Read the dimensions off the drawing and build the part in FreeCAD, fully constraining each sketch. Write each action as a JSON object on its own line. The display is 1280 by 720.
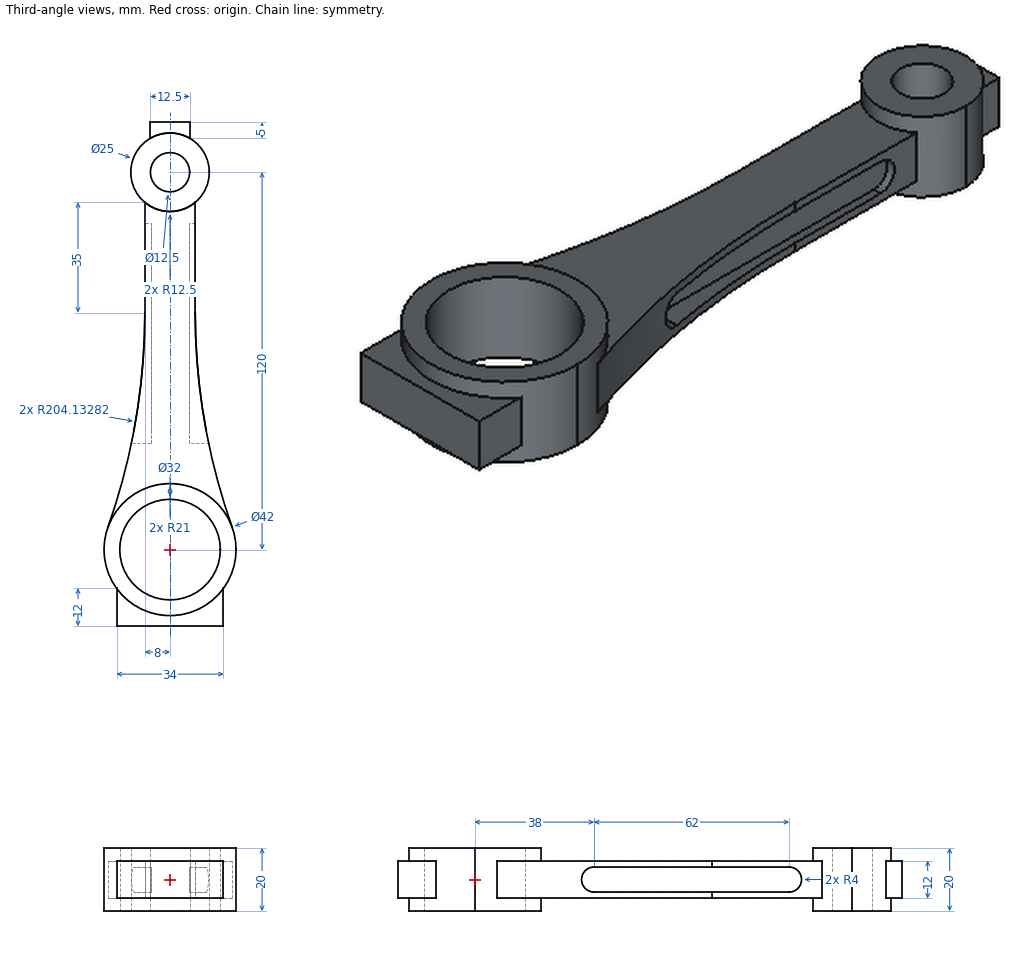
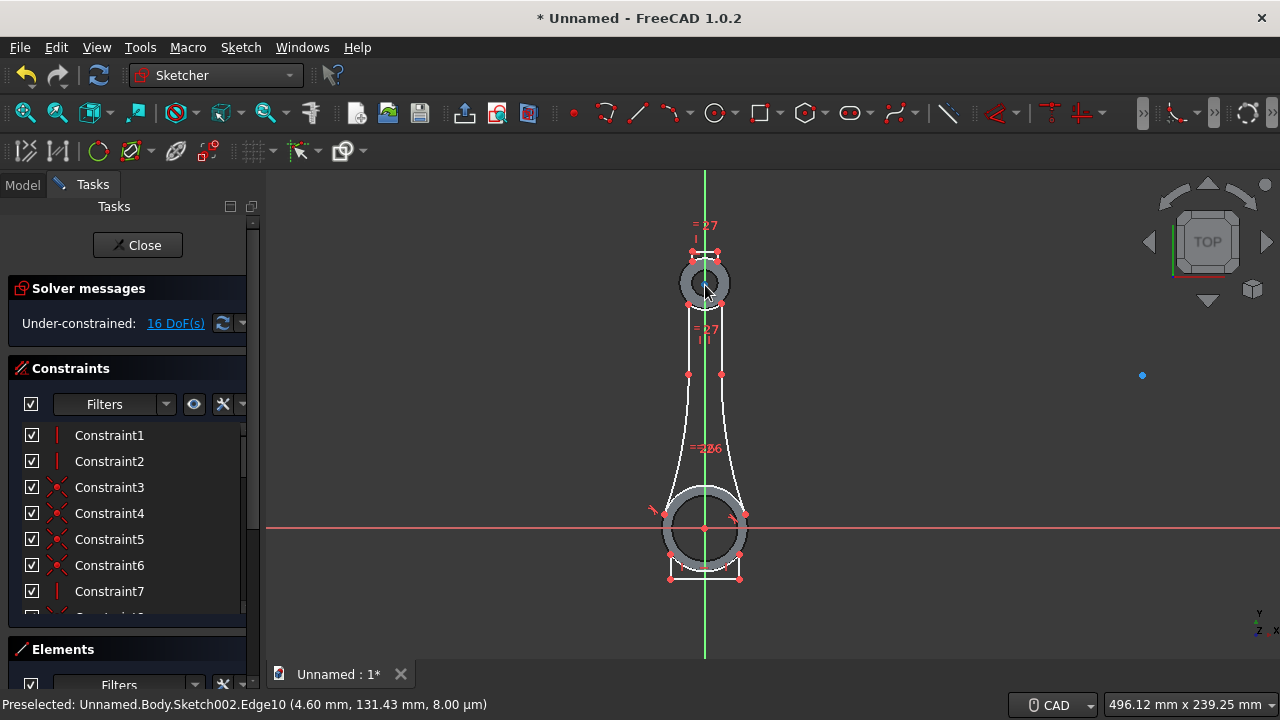
{"action": "left_click", "coordinate": [725, 491]}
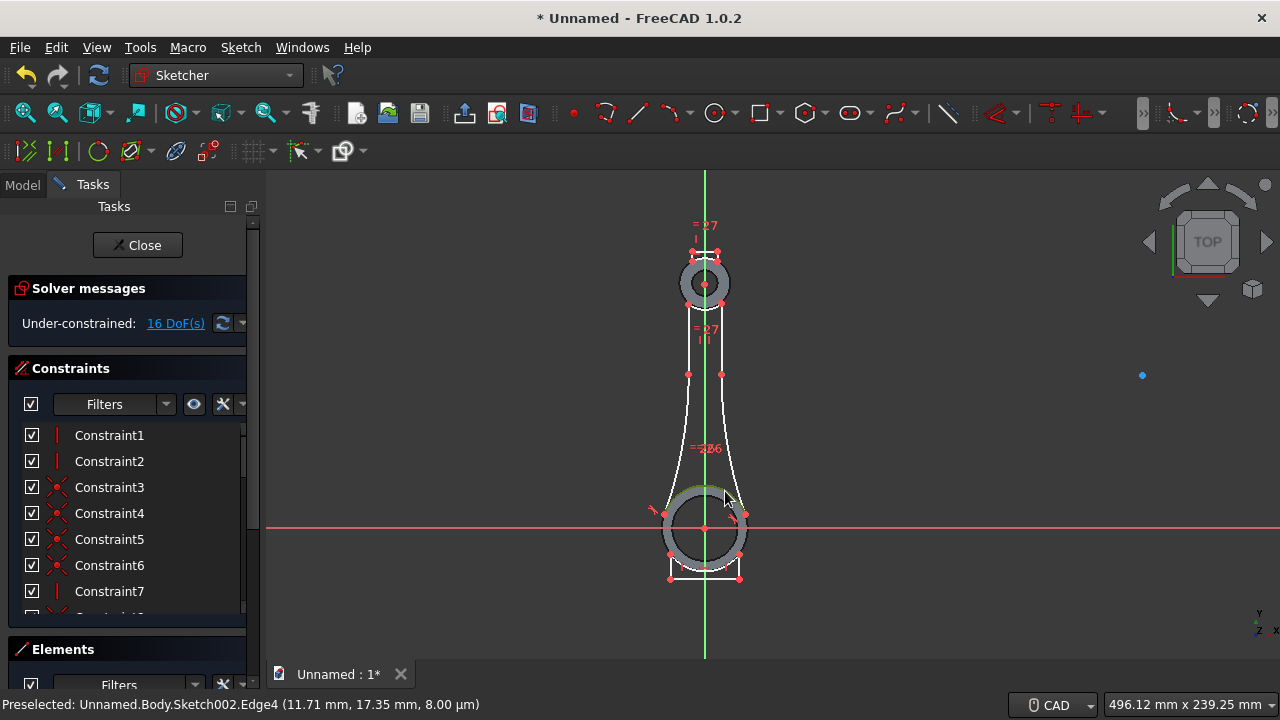
{"action": "scroll", "coordinate": [689, 569], "scroll_direction": "up", "scroll_amount": 2}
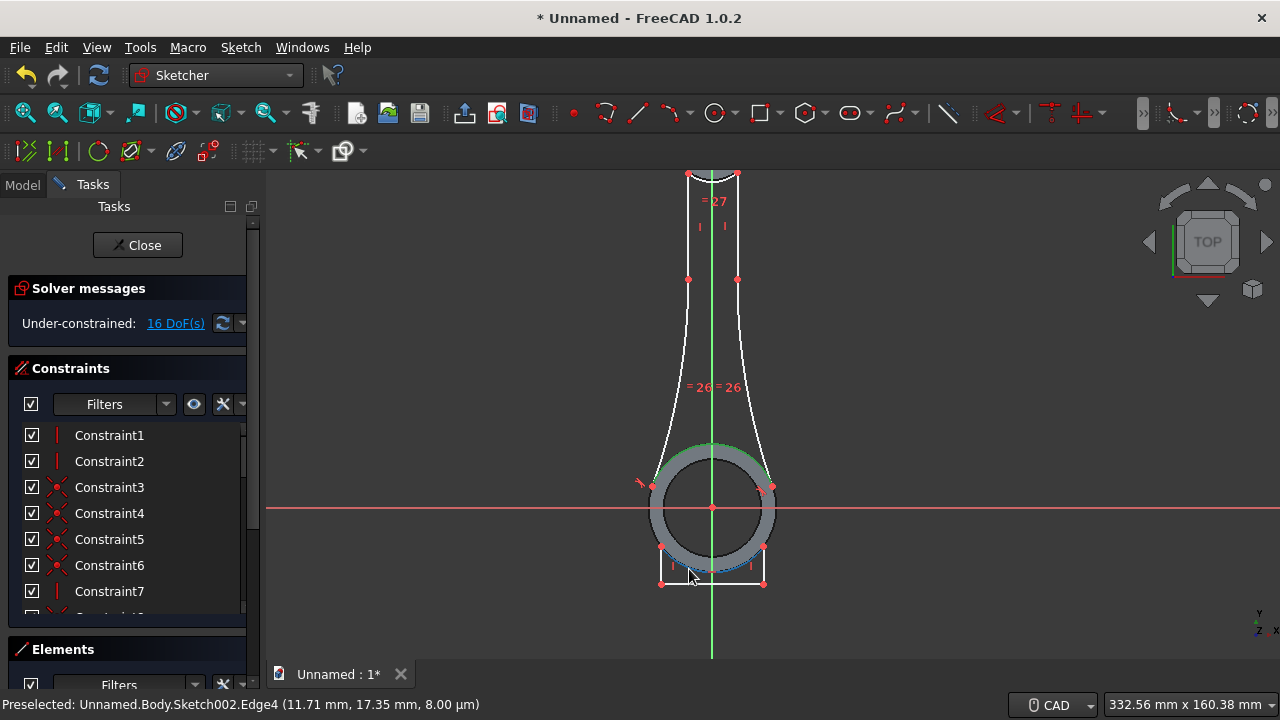
{"action": "left_click", "coordinate": [689, 568]}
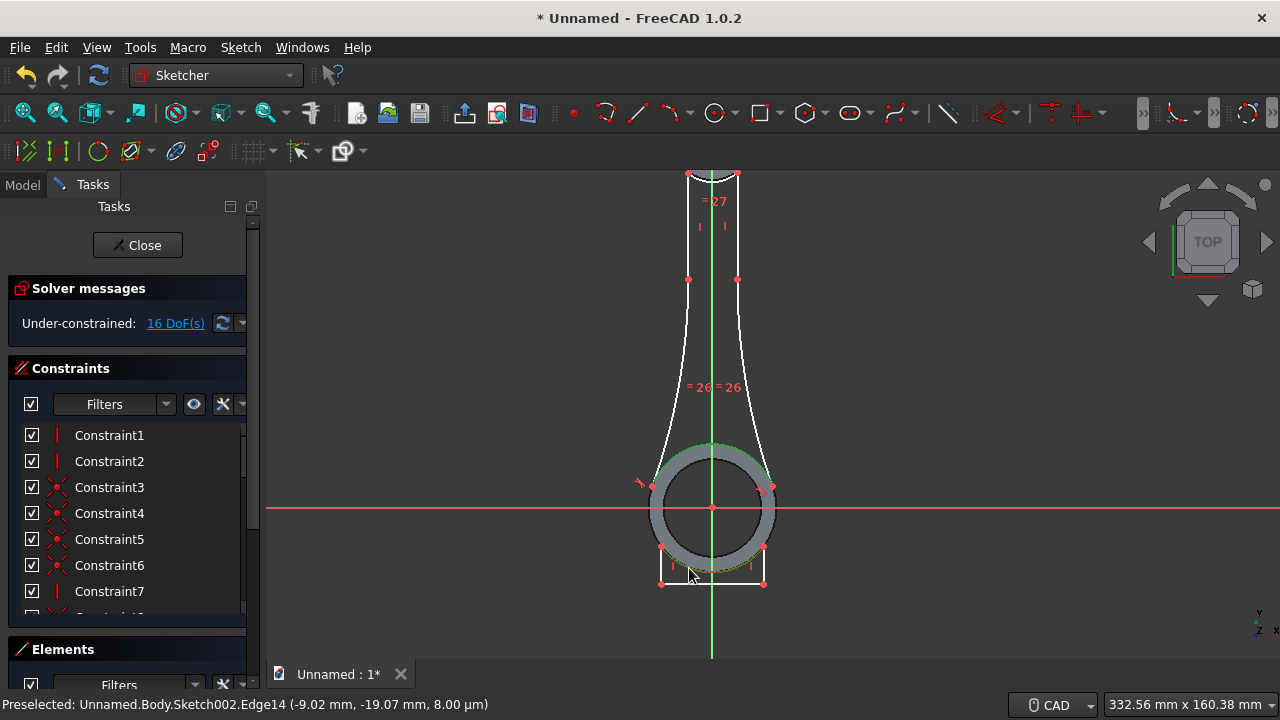
{"action": "key", "text": "e"}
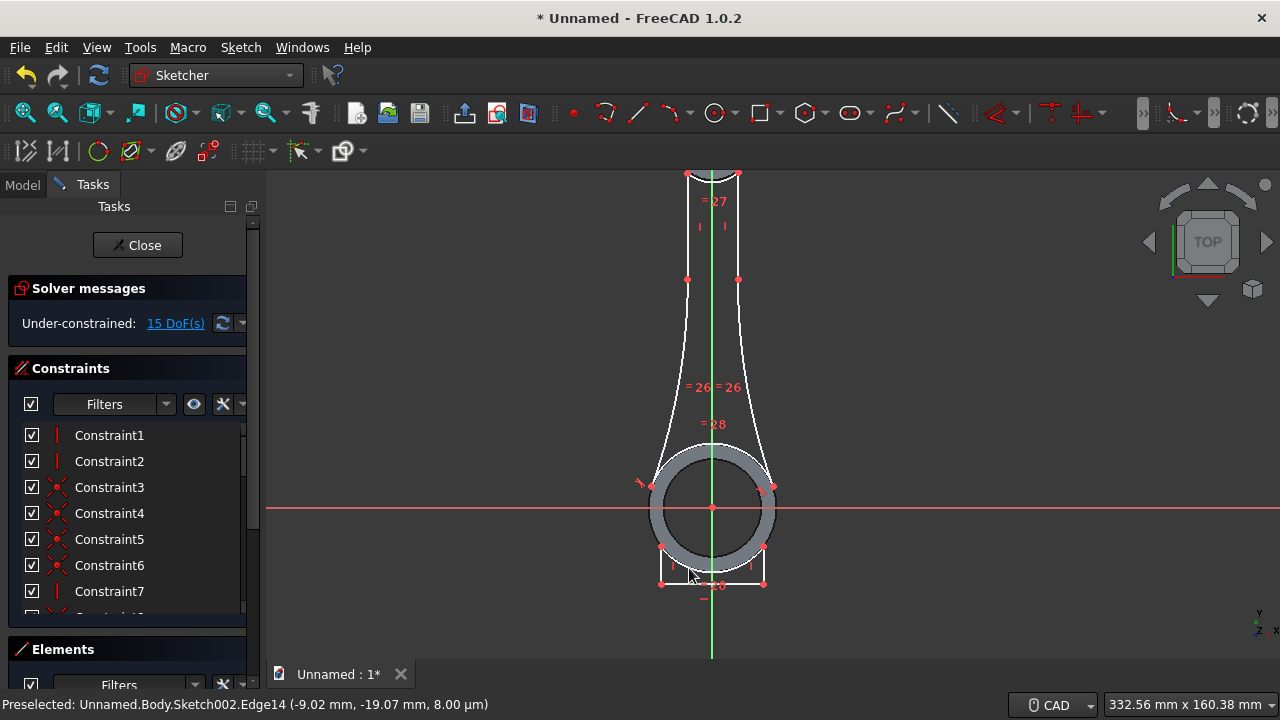
{"action": "scroll", "coordinate": [688, 570], "scroll_direction": "down", "scroll_amount": 2}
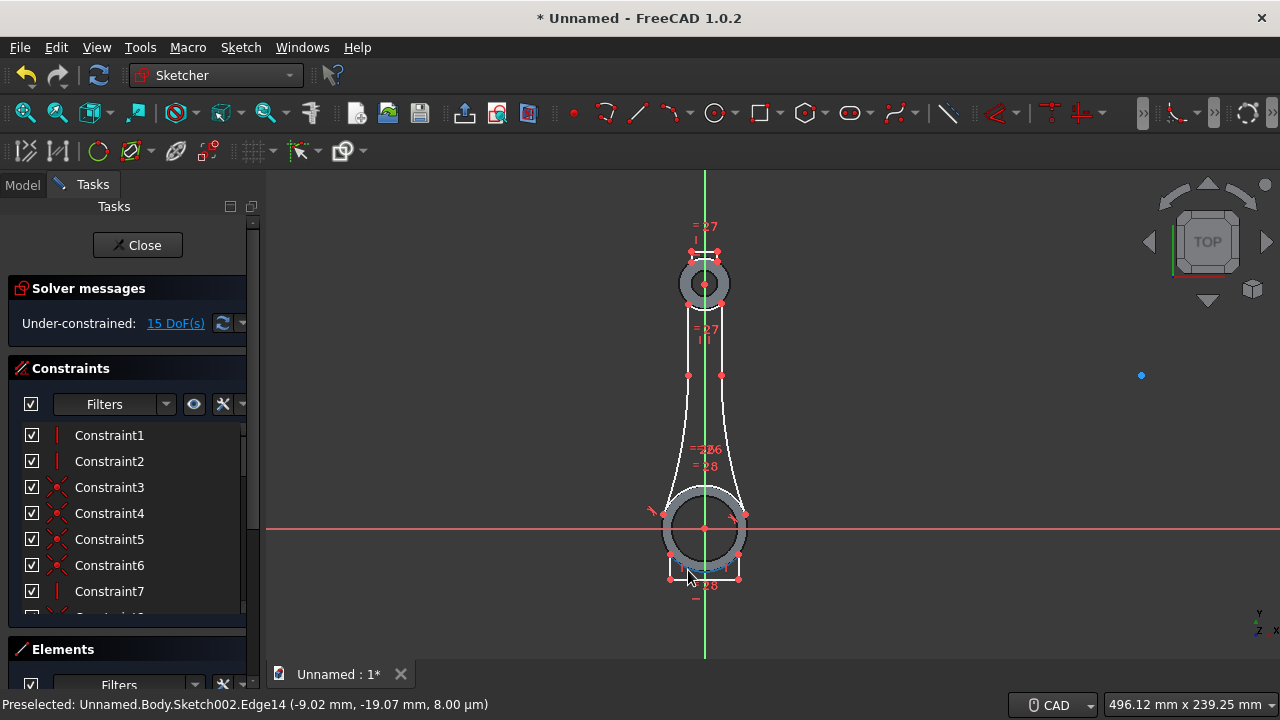
{"action": "left_click", "coordinate": [705, 285]}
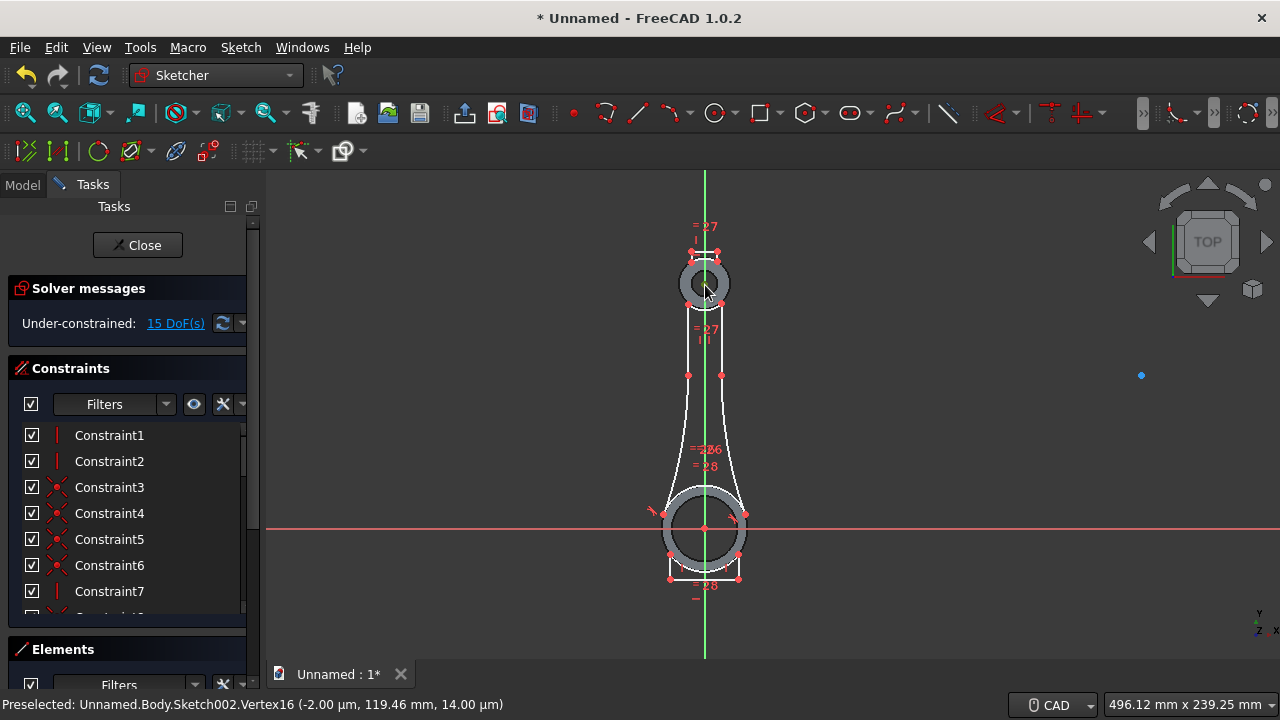
{"action": "left_click", "coordinate": [705, 507]}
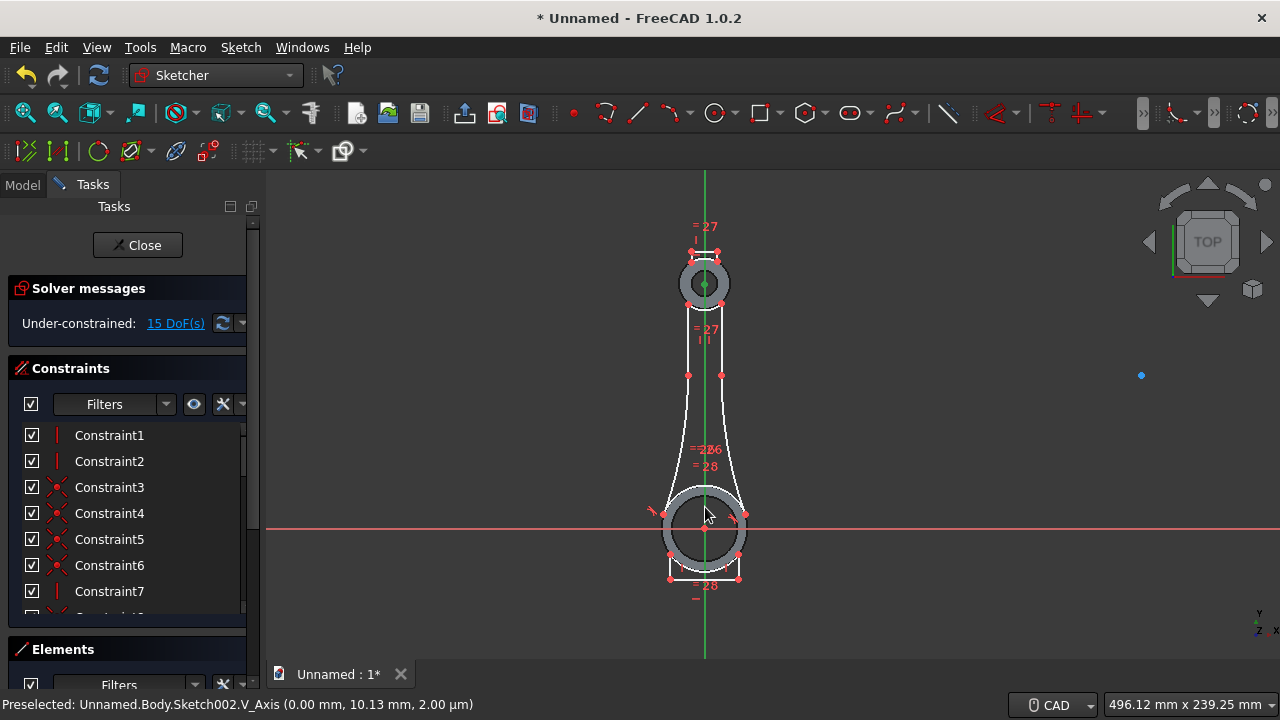
{"action": "key", "text": "c"}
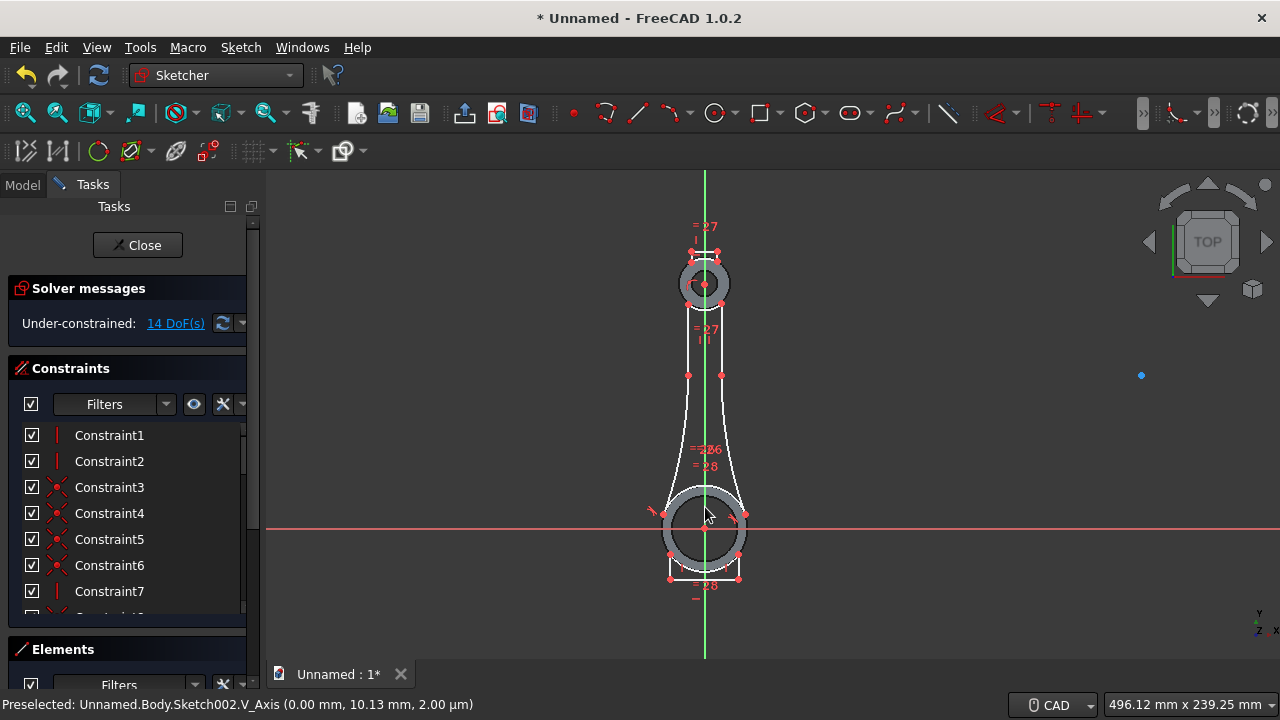
{"action": "left_click", "coordinate": [688, 375]}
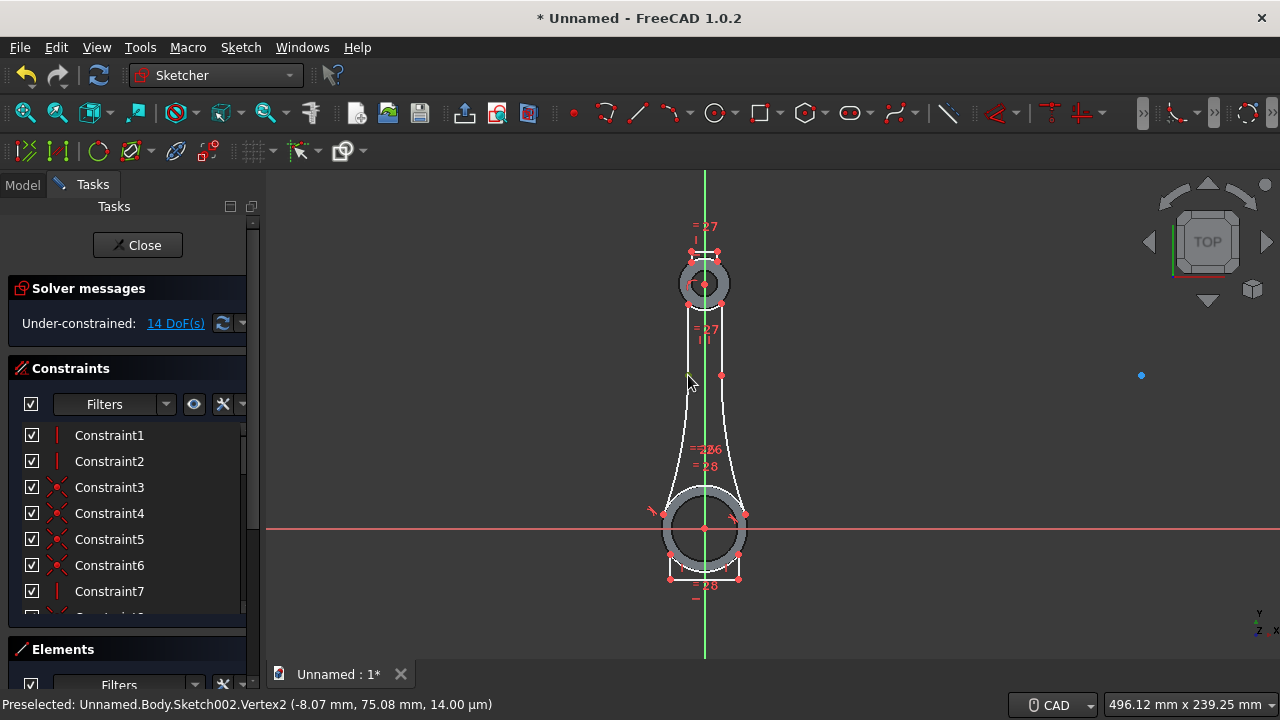
{"action": "left_click", "coordinate": [722, 375]}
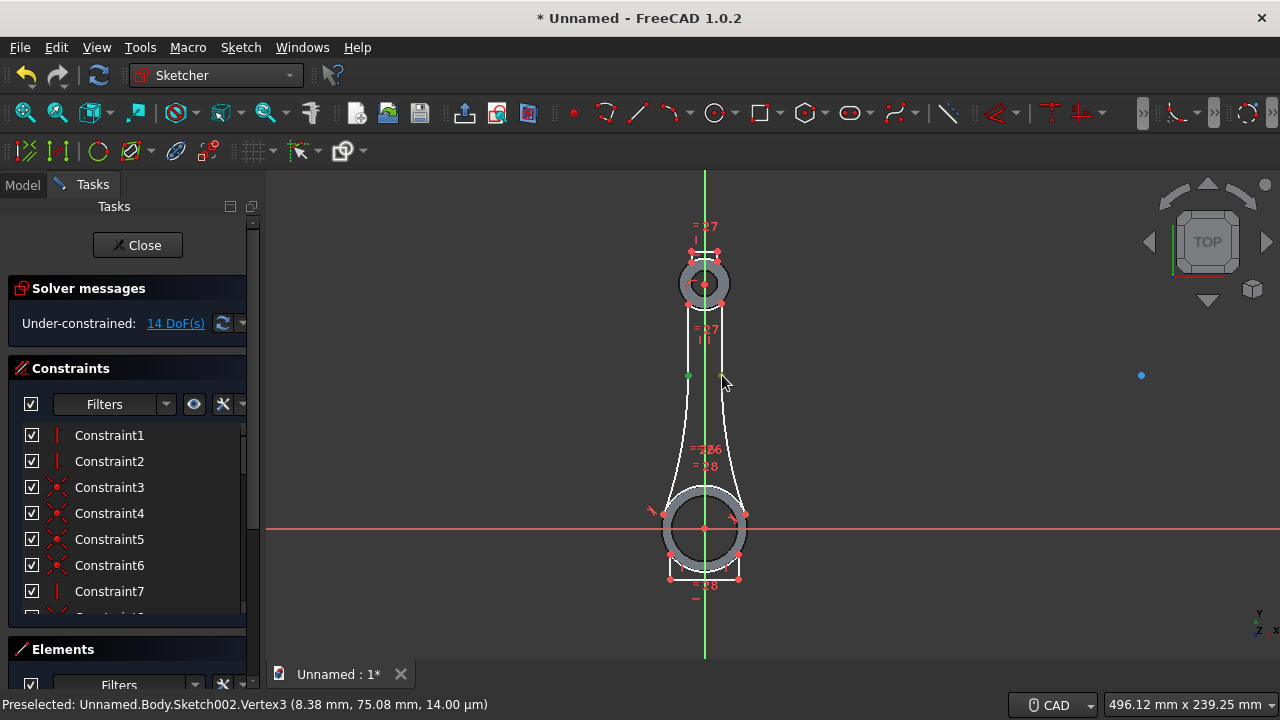
{"action": "left_click", "coordinate": [705, 507]}